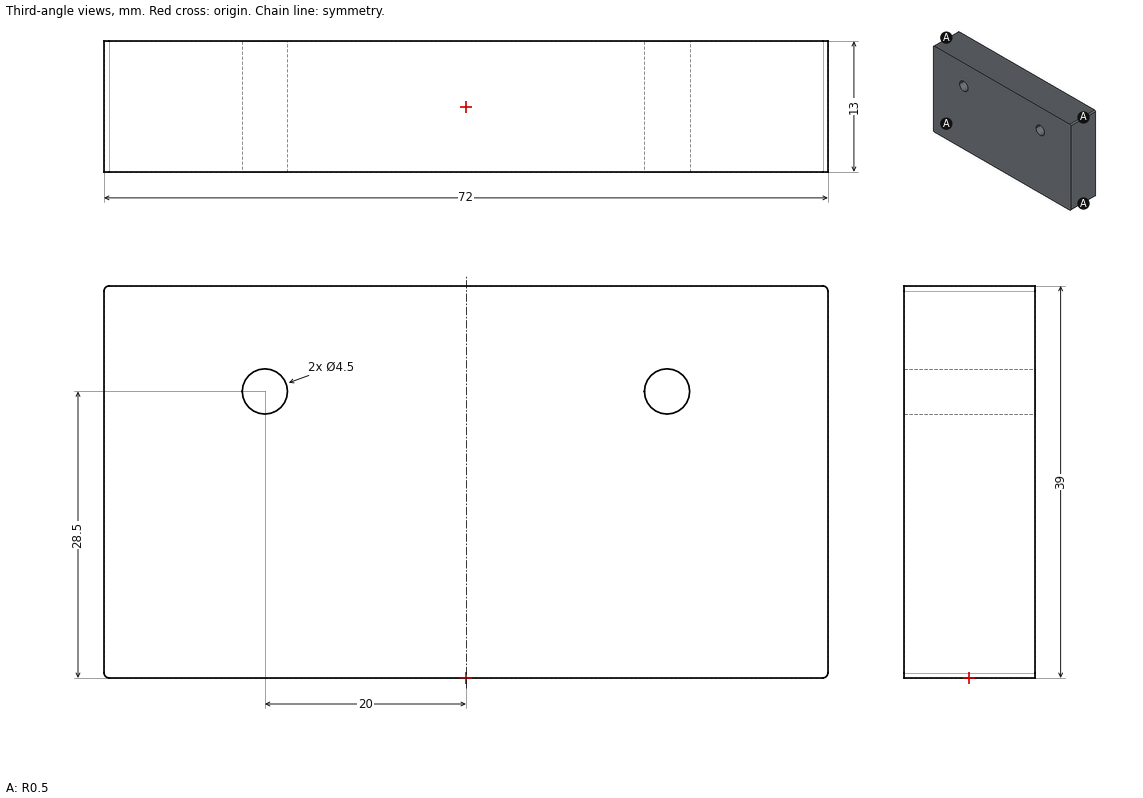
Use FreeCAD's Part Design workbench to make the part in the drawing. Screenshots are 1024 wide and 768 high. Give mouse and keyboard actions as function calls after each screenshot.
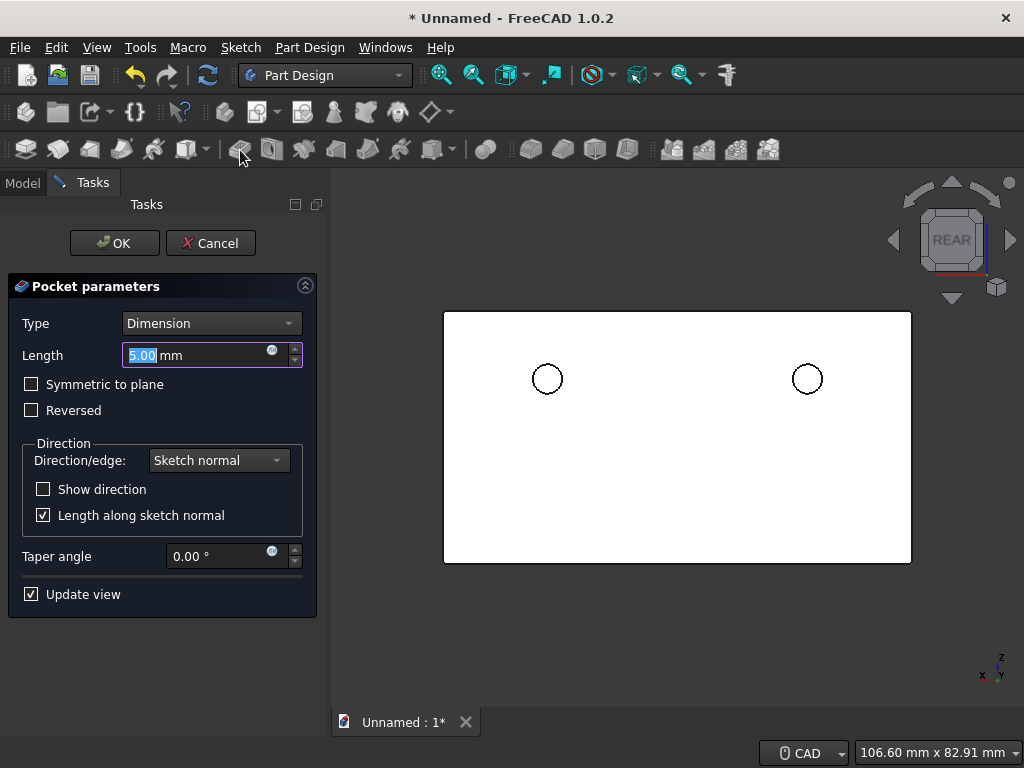
click(212, 324)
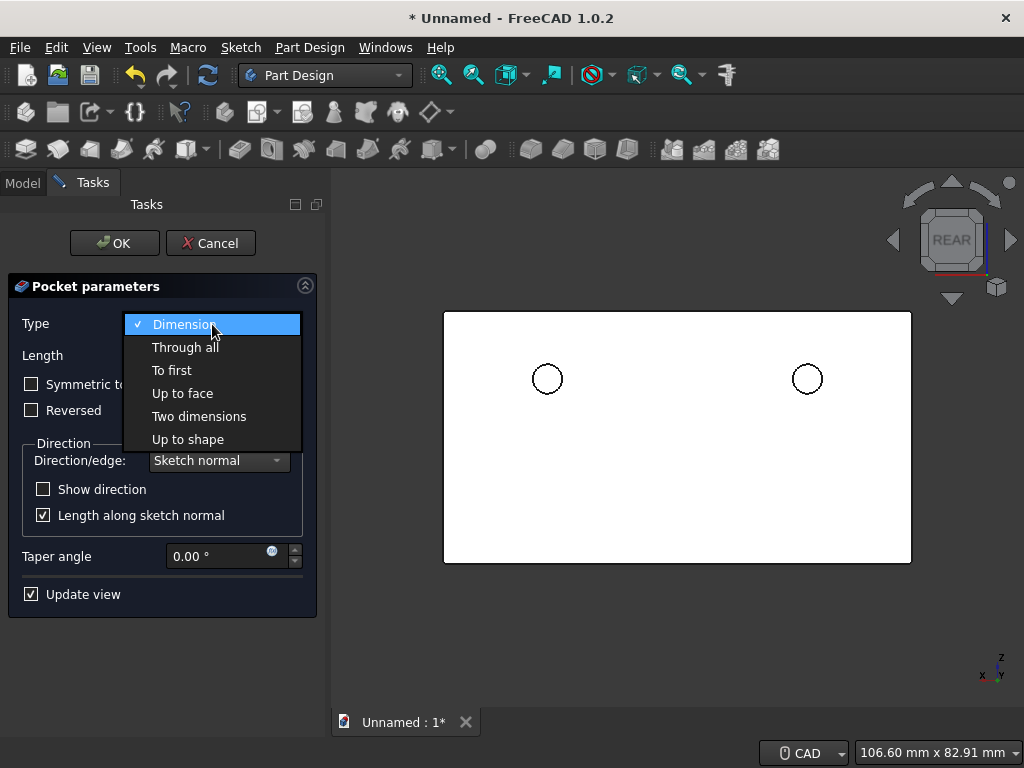
click(212, 348)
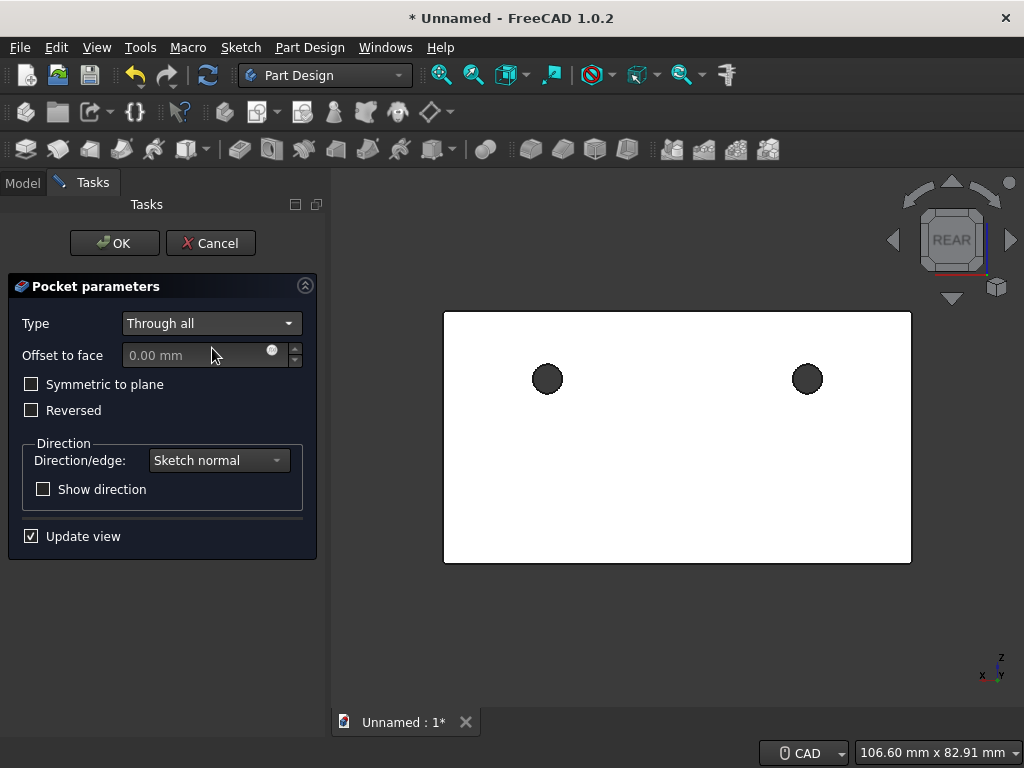
click(115, 243)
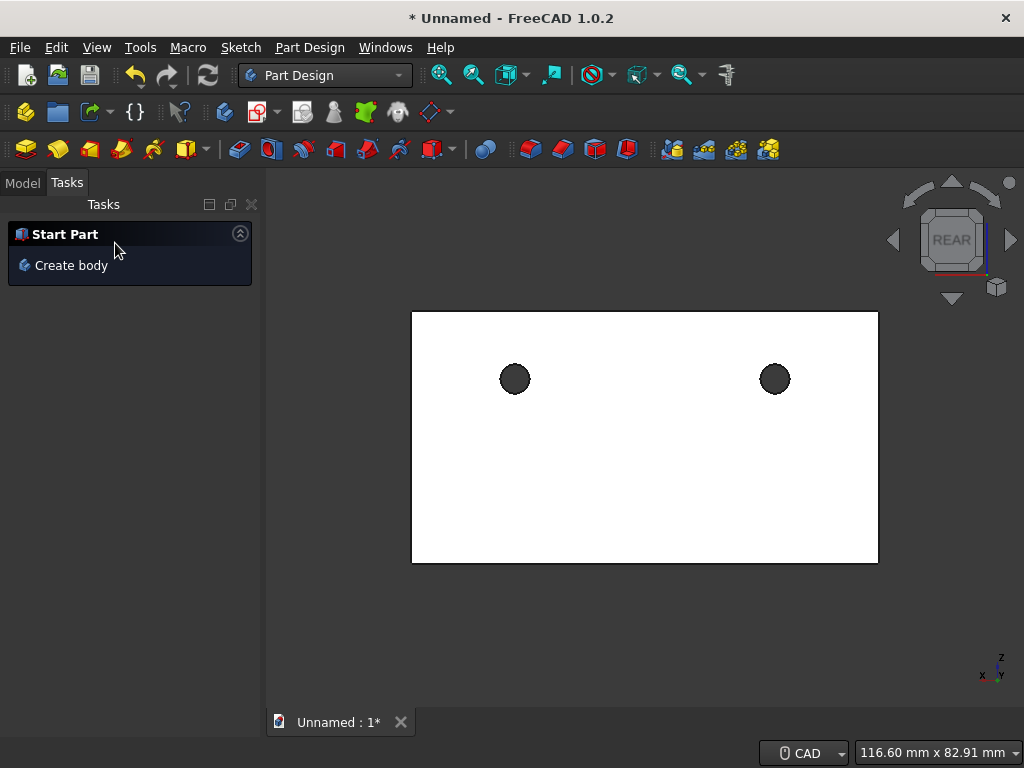
key(0)